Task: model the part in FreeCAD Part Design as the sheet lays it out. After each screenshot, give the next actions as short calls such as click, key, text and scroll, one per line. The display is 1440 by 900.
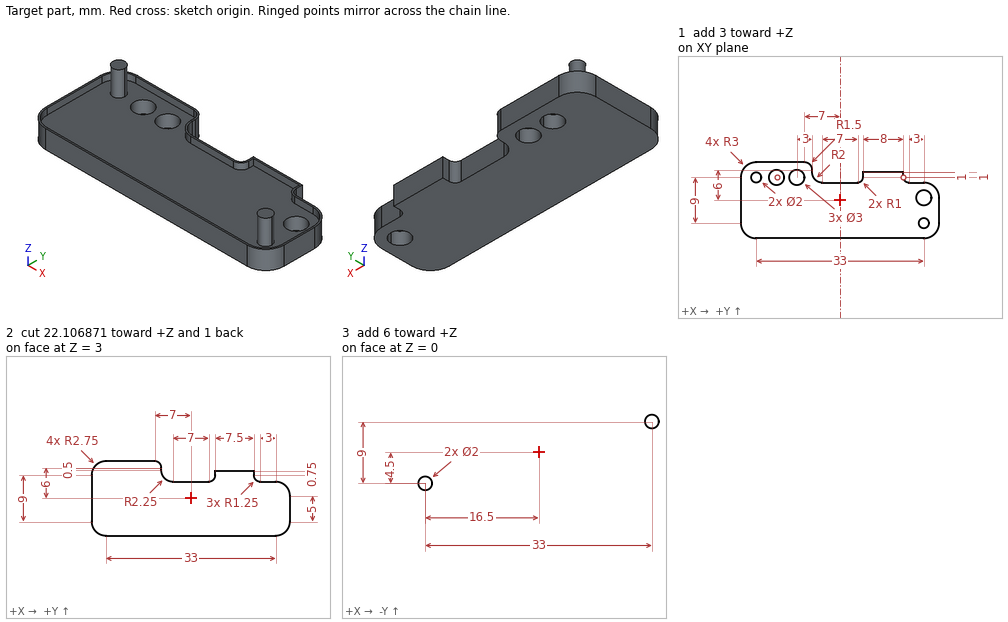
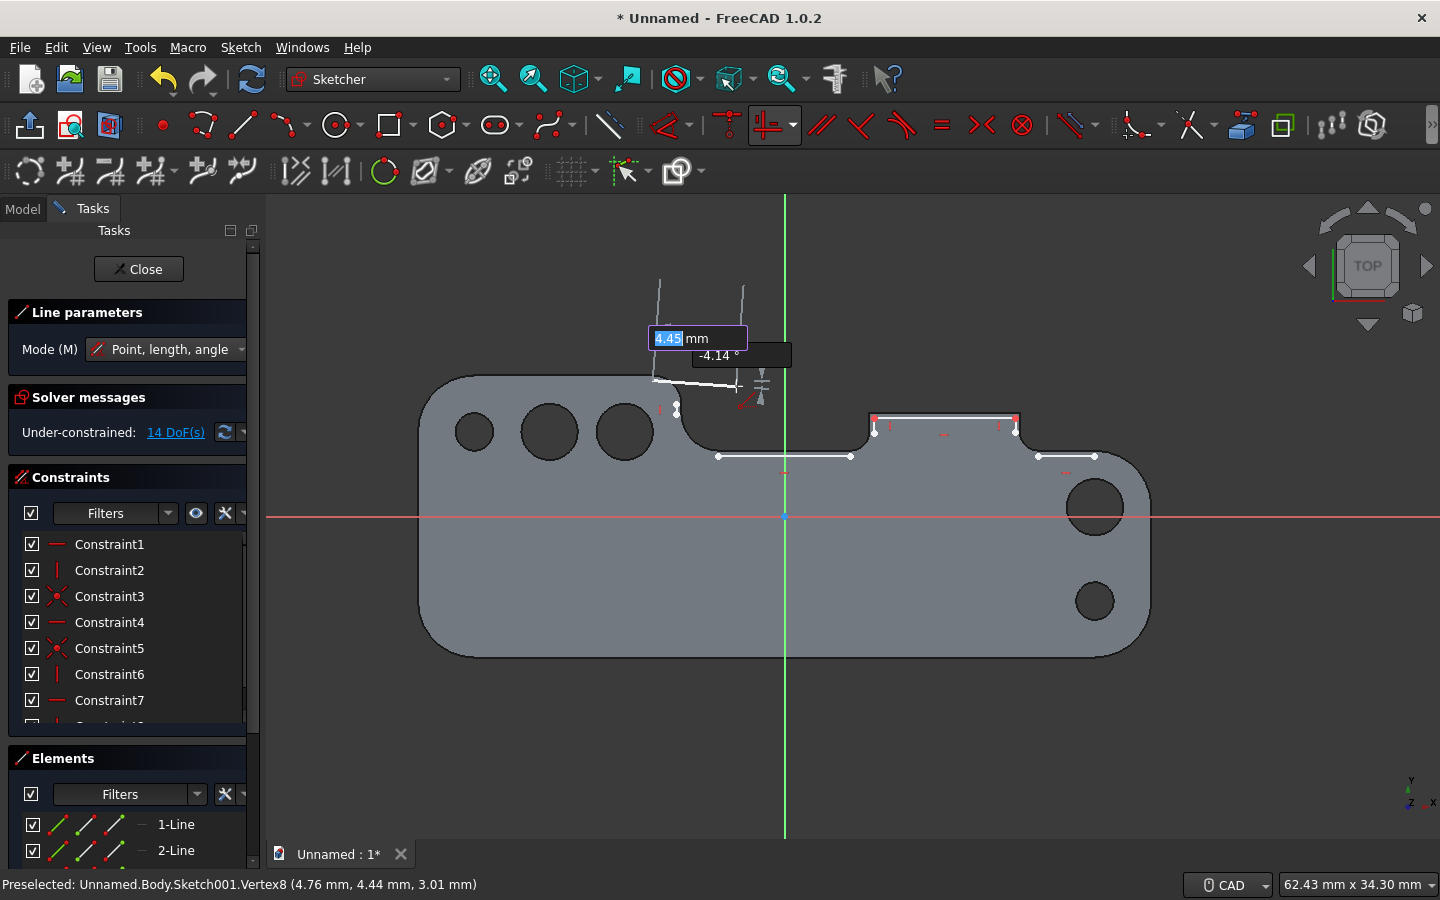
click(474, 380)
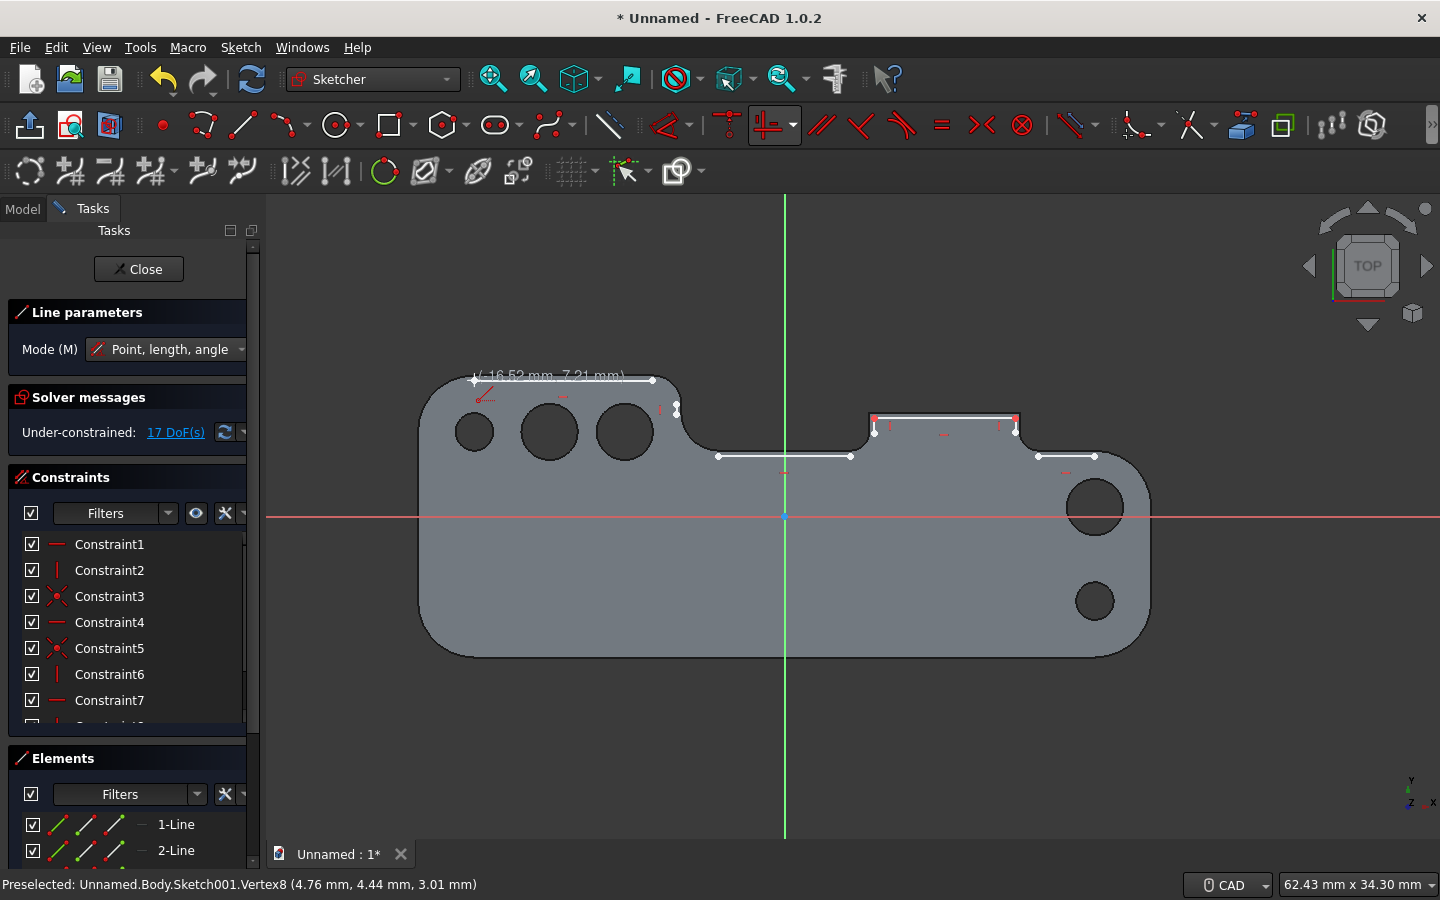
click(423, 432)
click(423, 601)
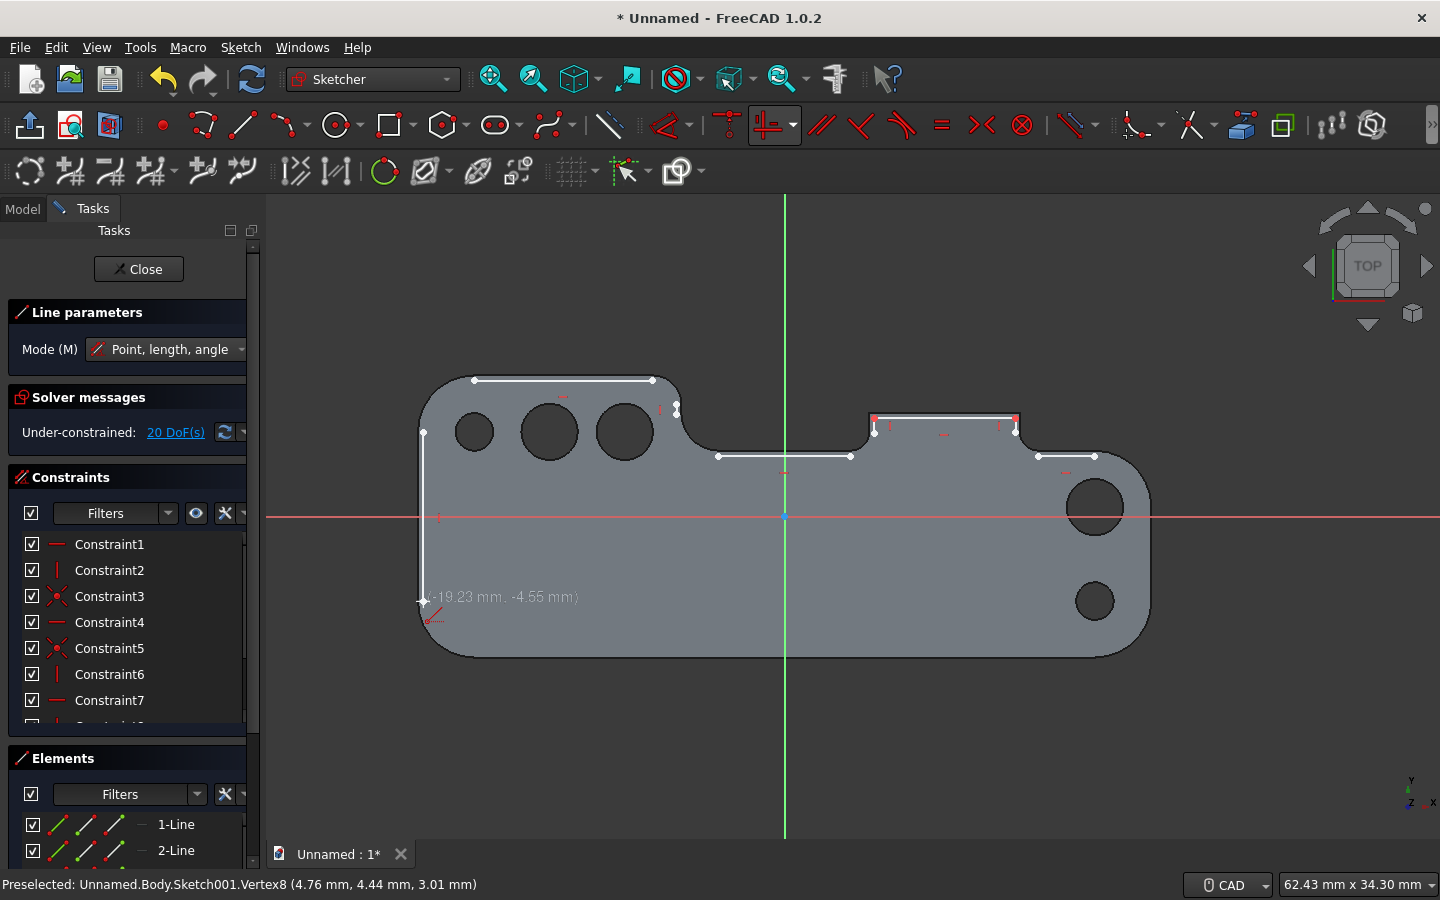
click(474, 653)
click(1095, 653)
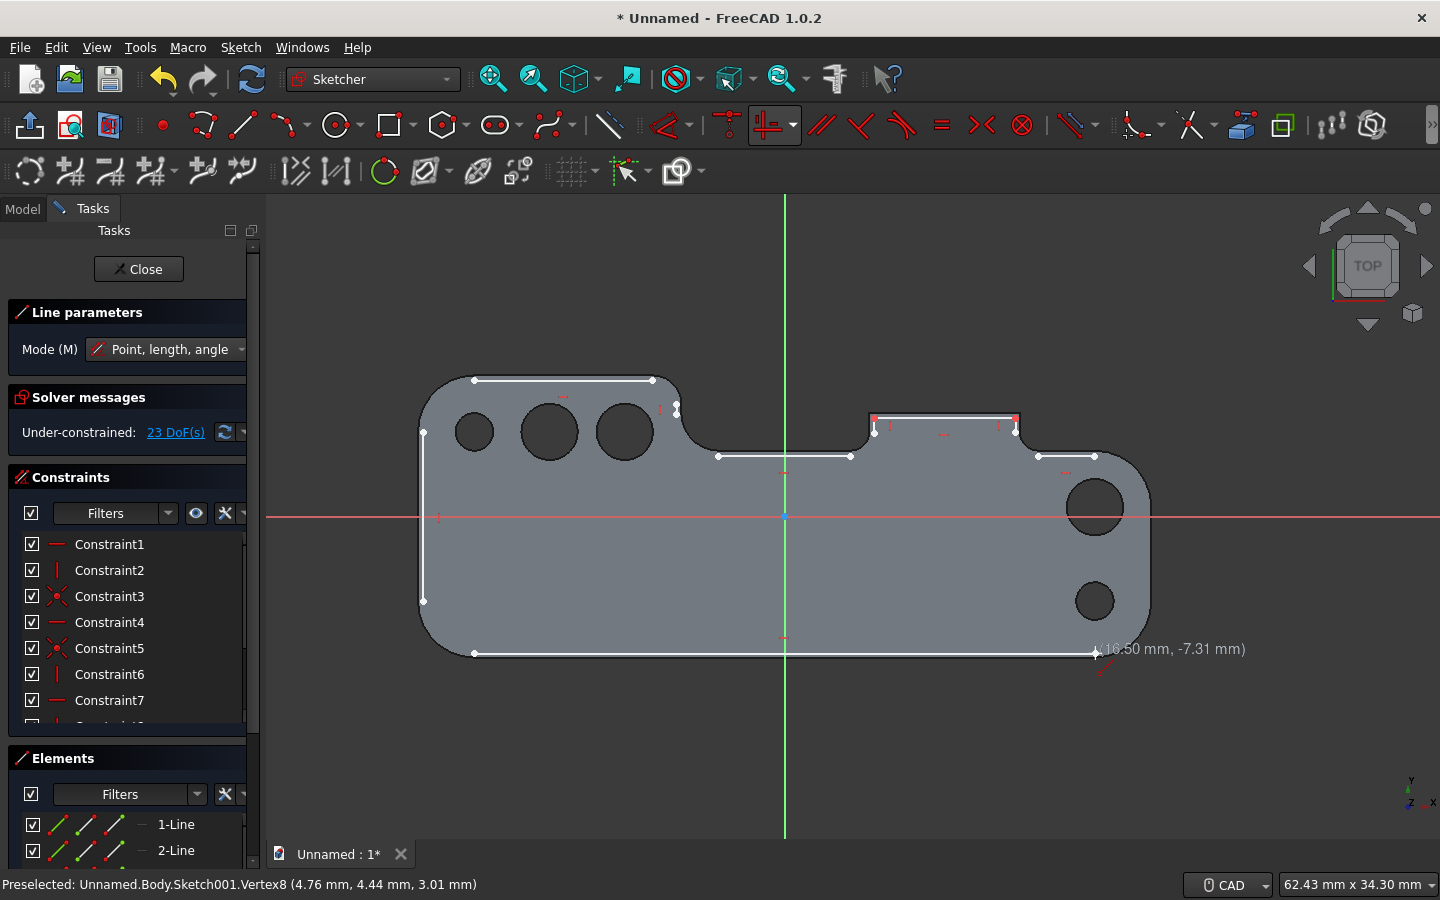
click(1147, 601)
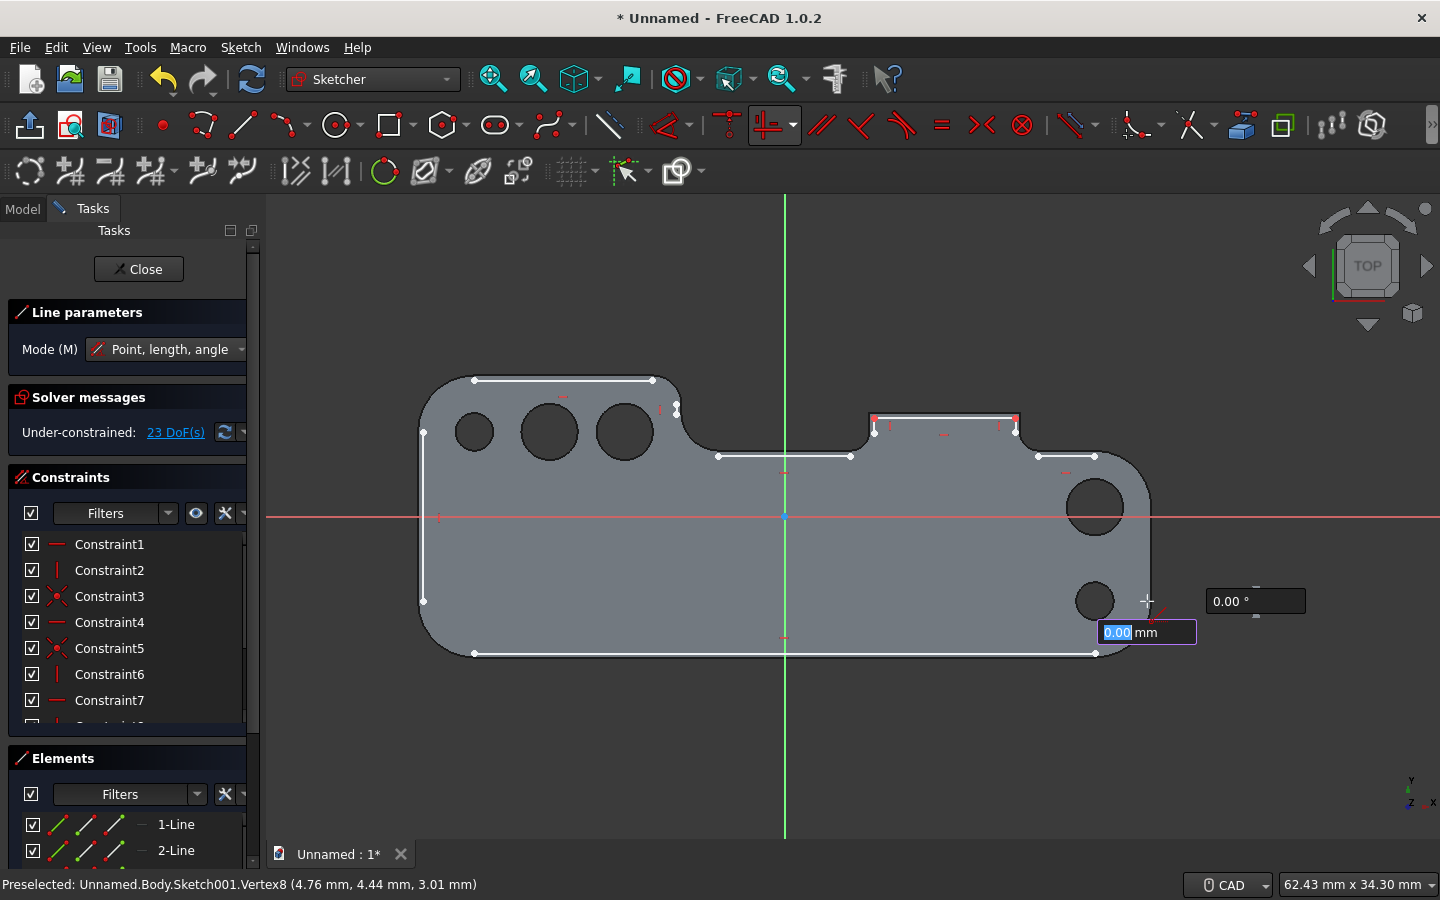
scroll(1147, 507, up, 3)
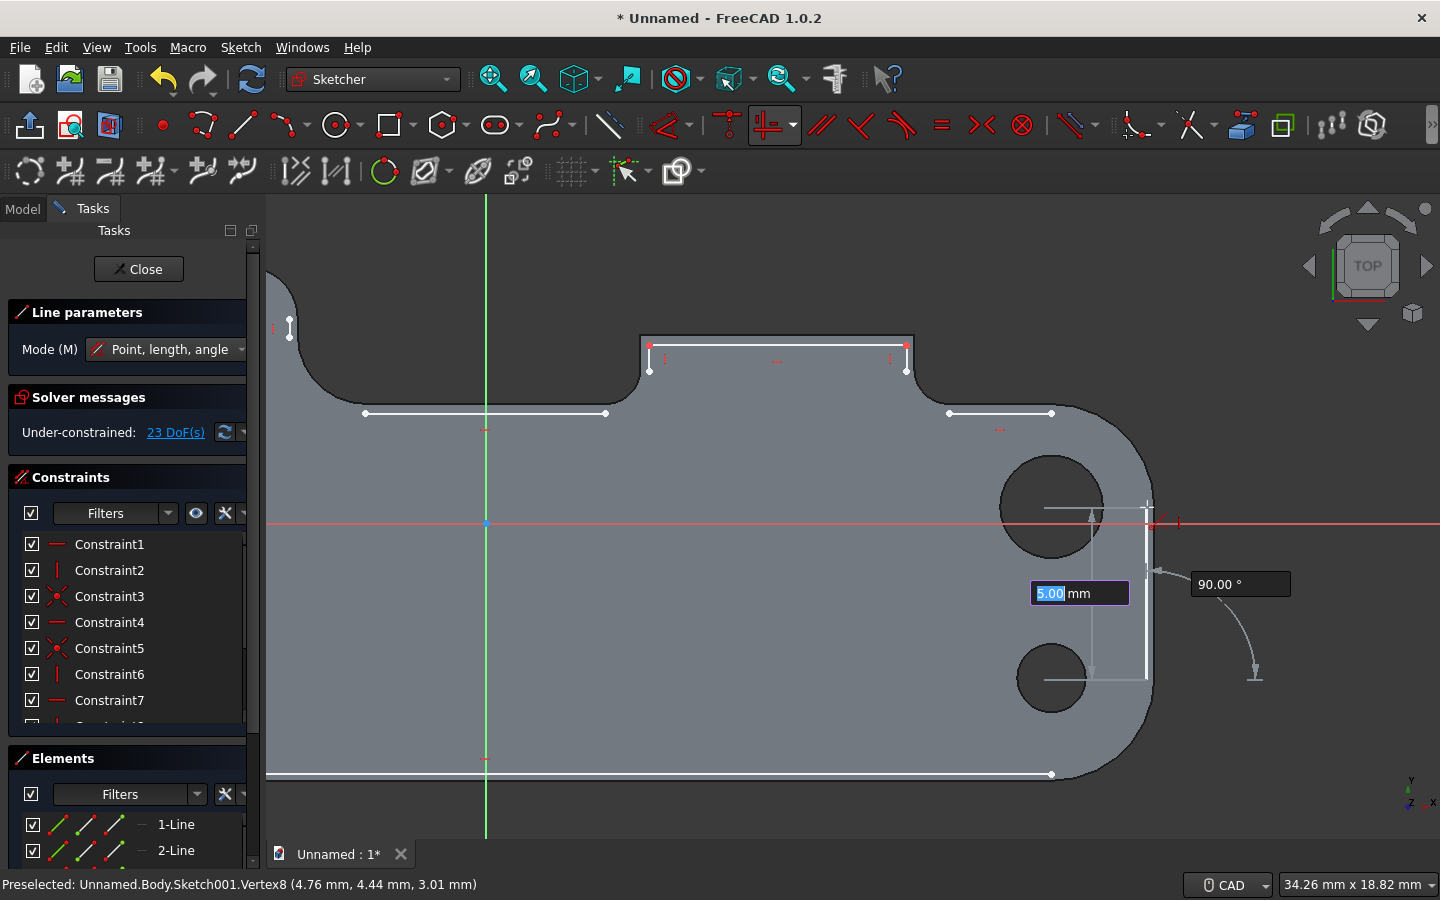
click(1146, 507)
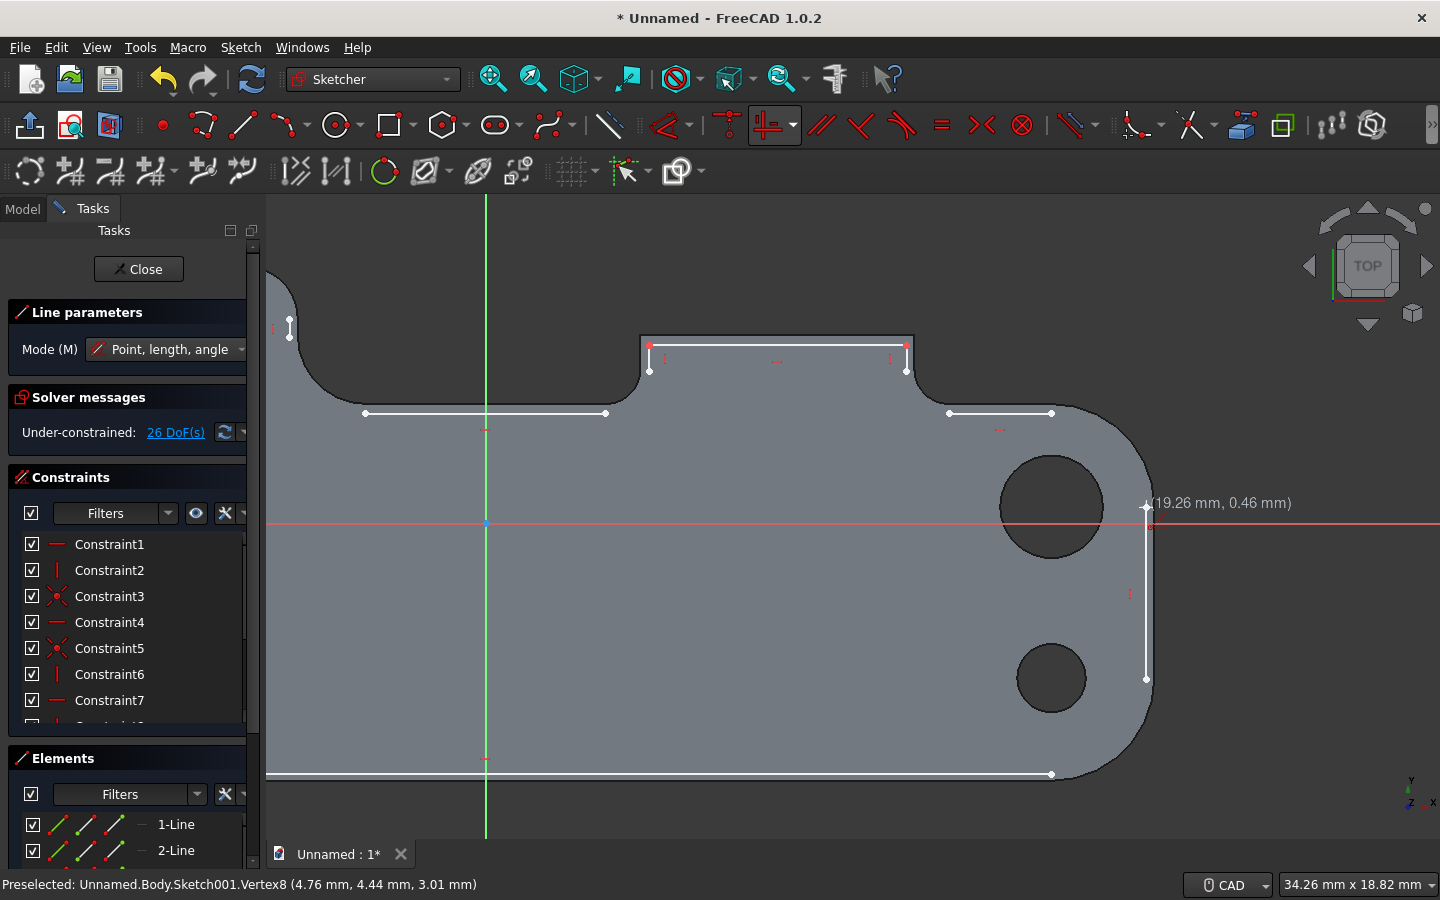
click(284, 126)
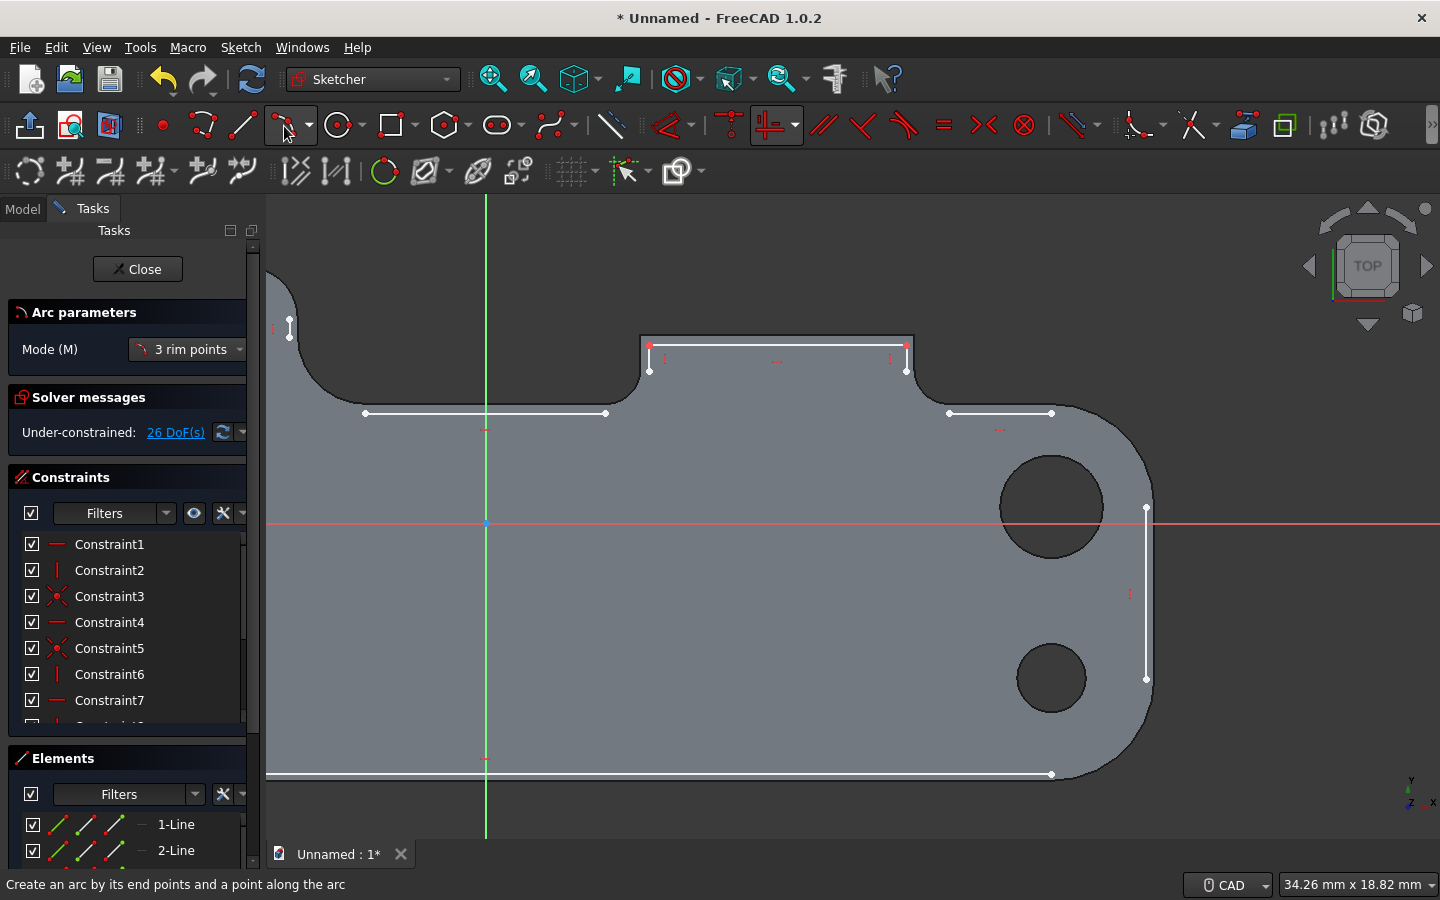
click(949, 414)